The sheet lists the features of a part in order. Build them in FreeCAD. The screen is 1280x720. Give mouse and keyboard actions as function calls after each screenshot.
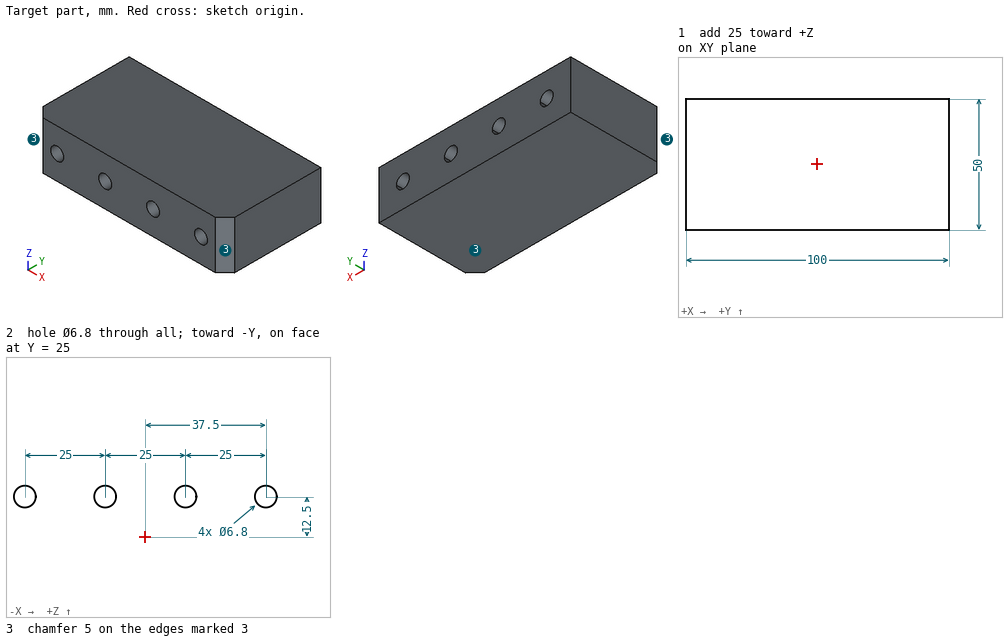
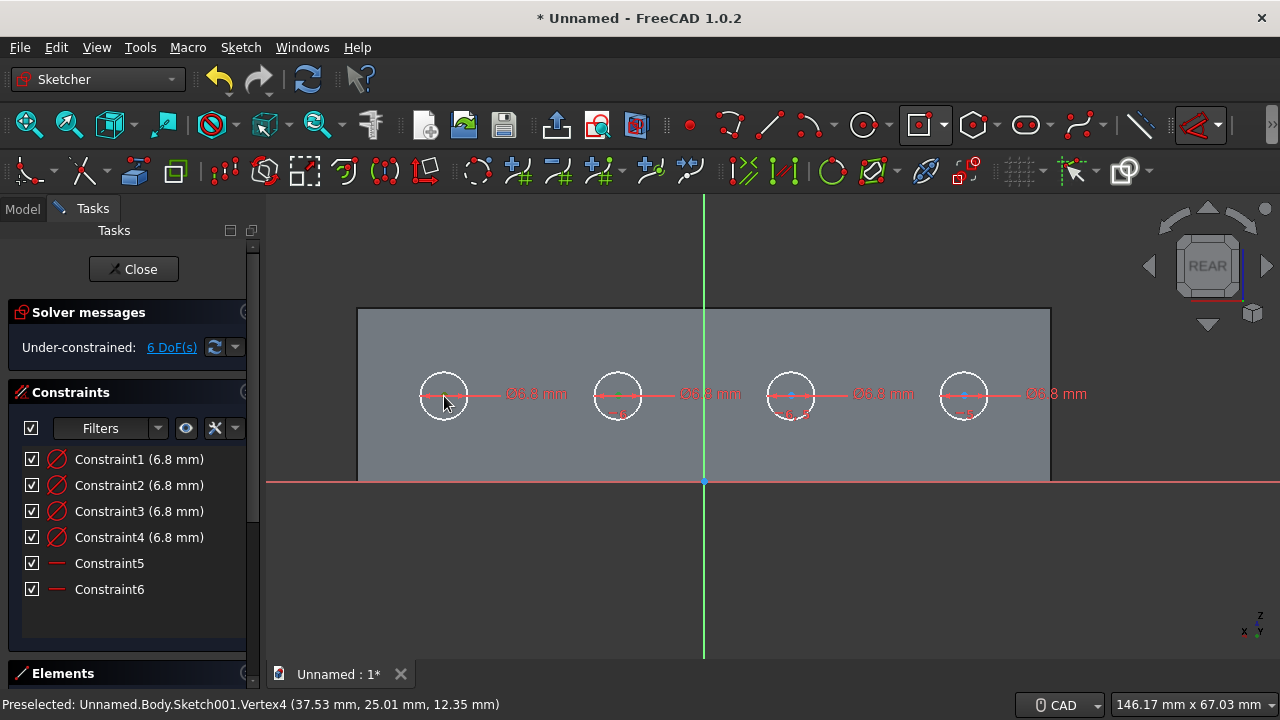
key(h)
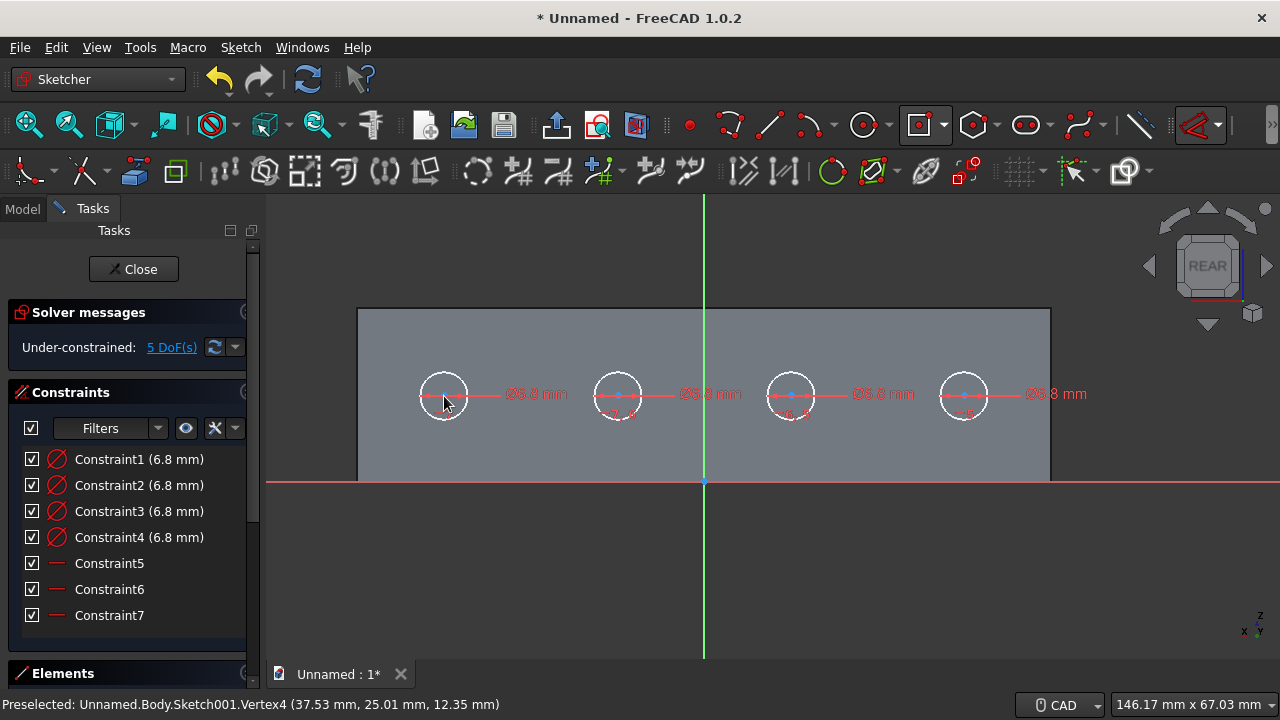
click(1194, 126)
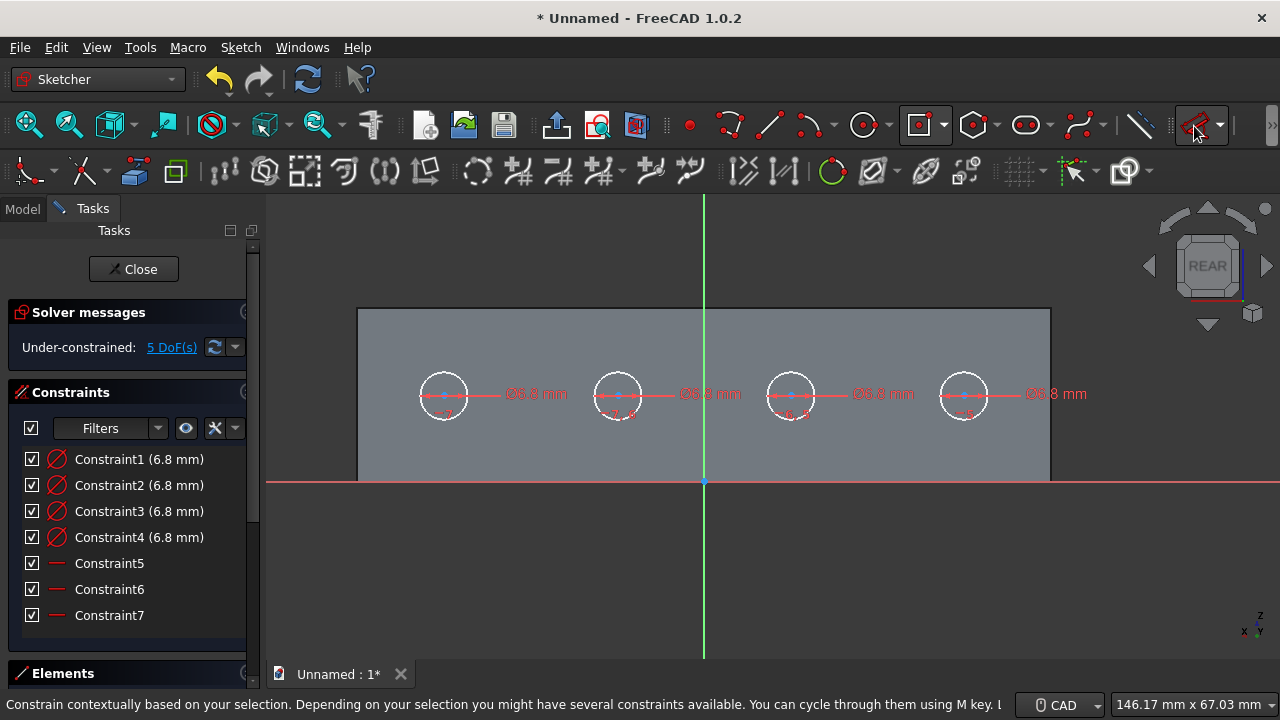
click(964, 396)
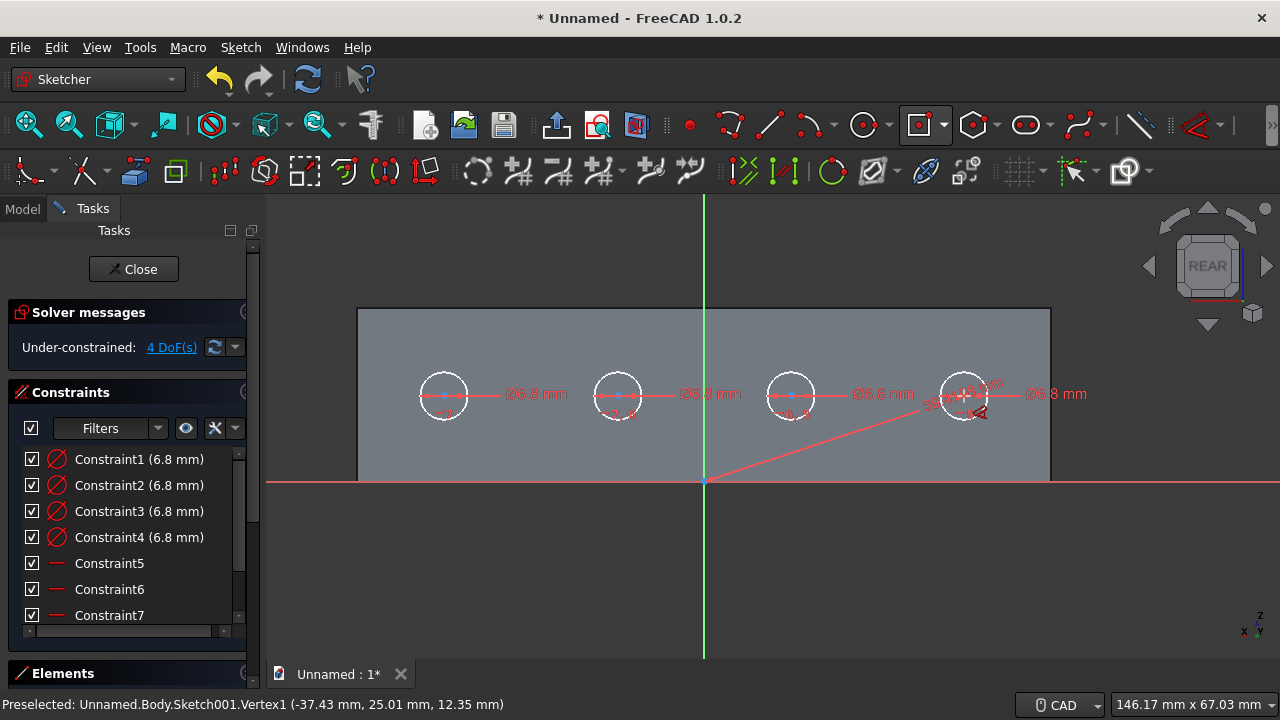
click(791, 396)
click(877, 362)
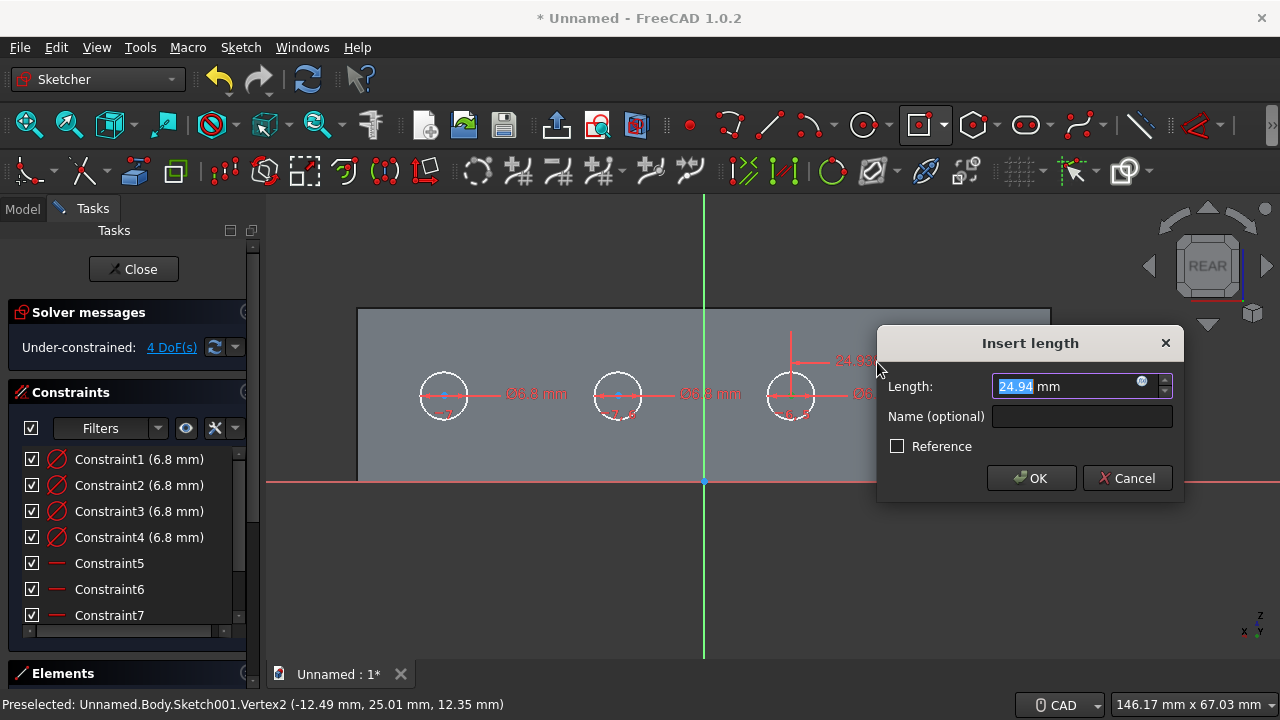
text(25)
key(Return)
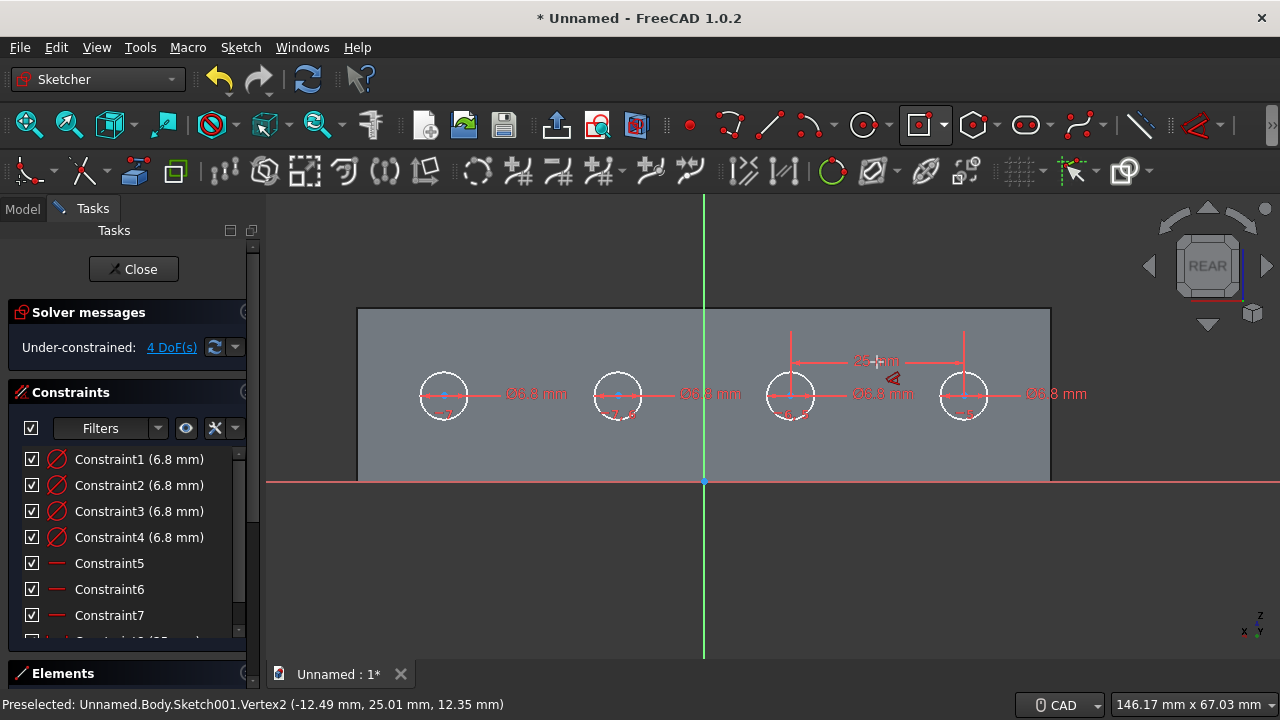
click(791, 396)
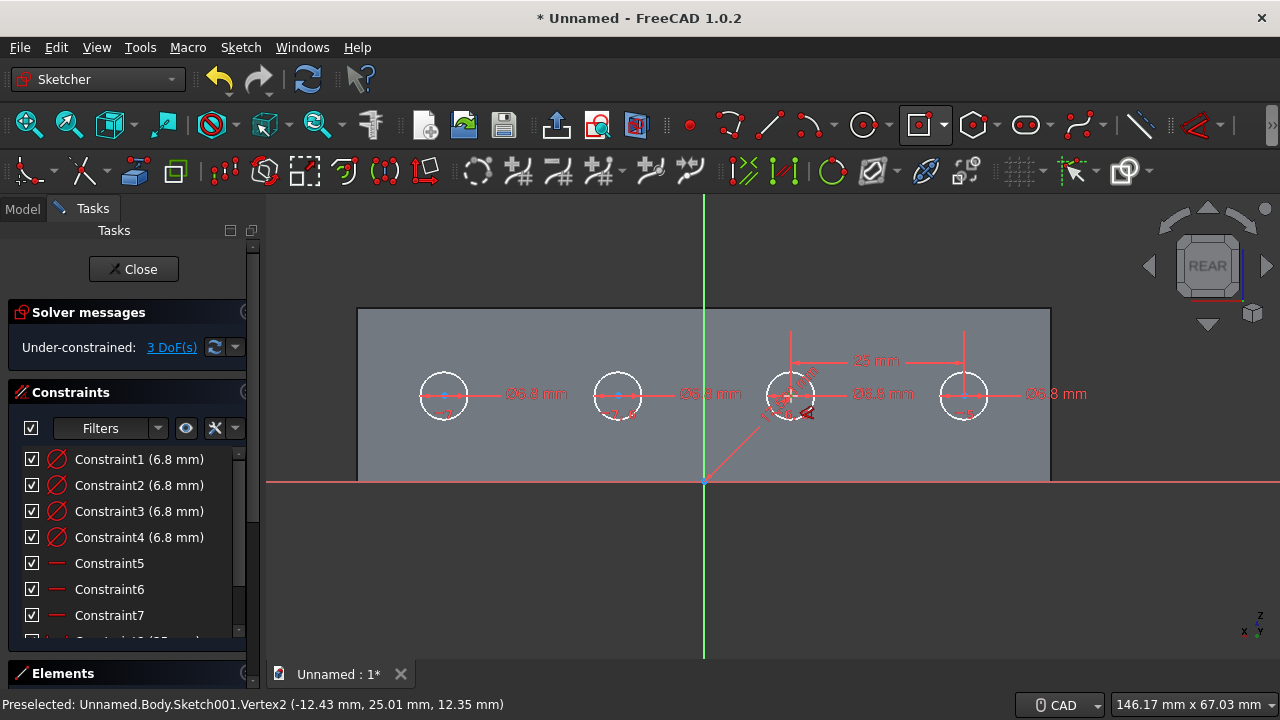
click(618, 396)
click(665, 362)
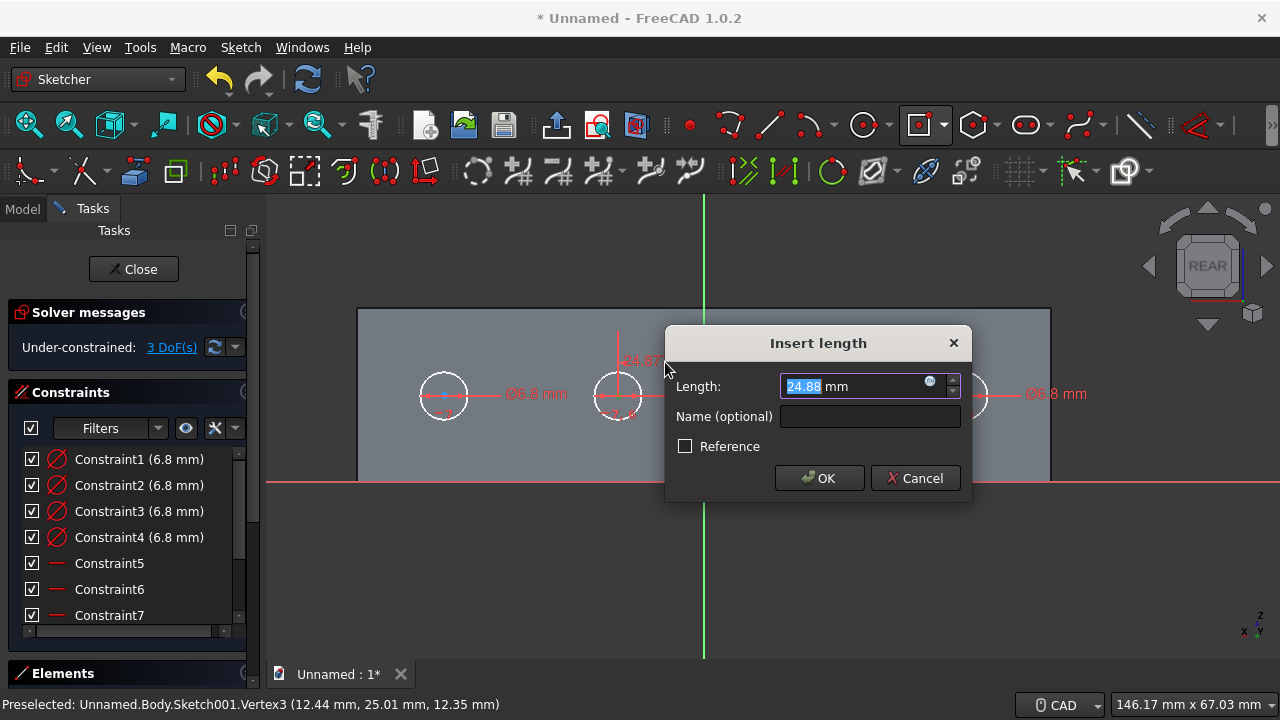
text(25)
key(Return)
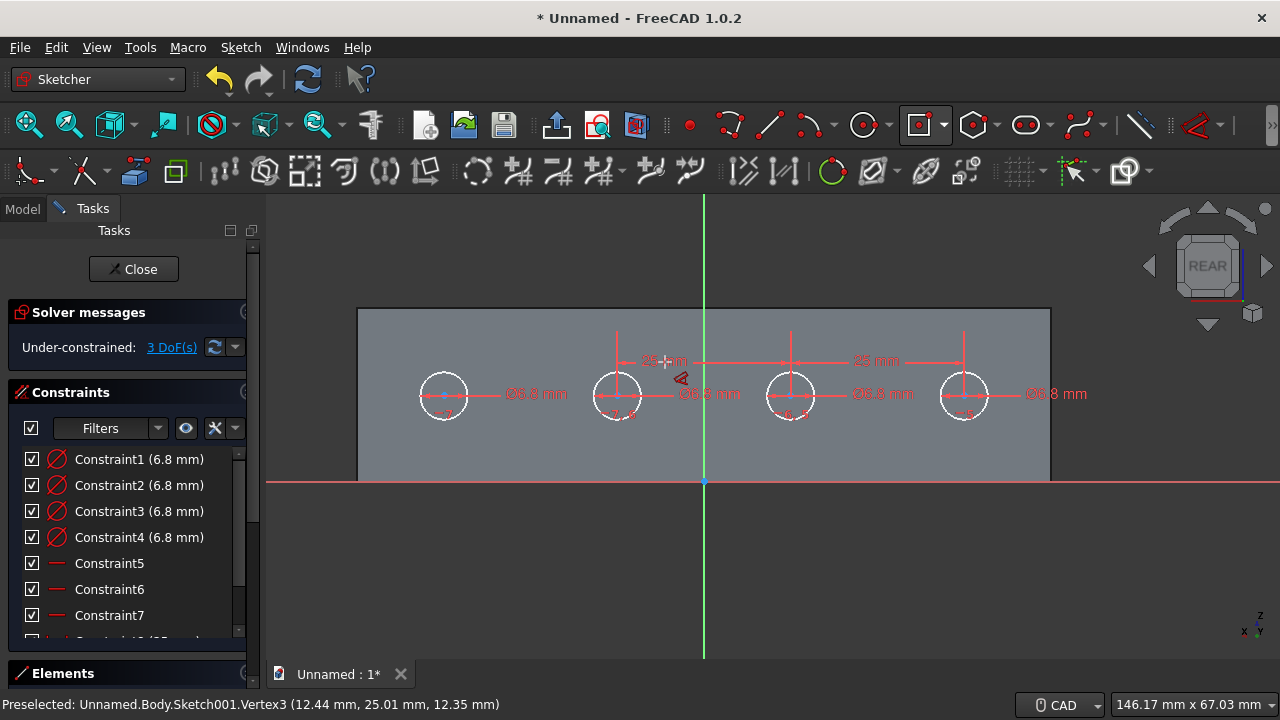
click(617, 396)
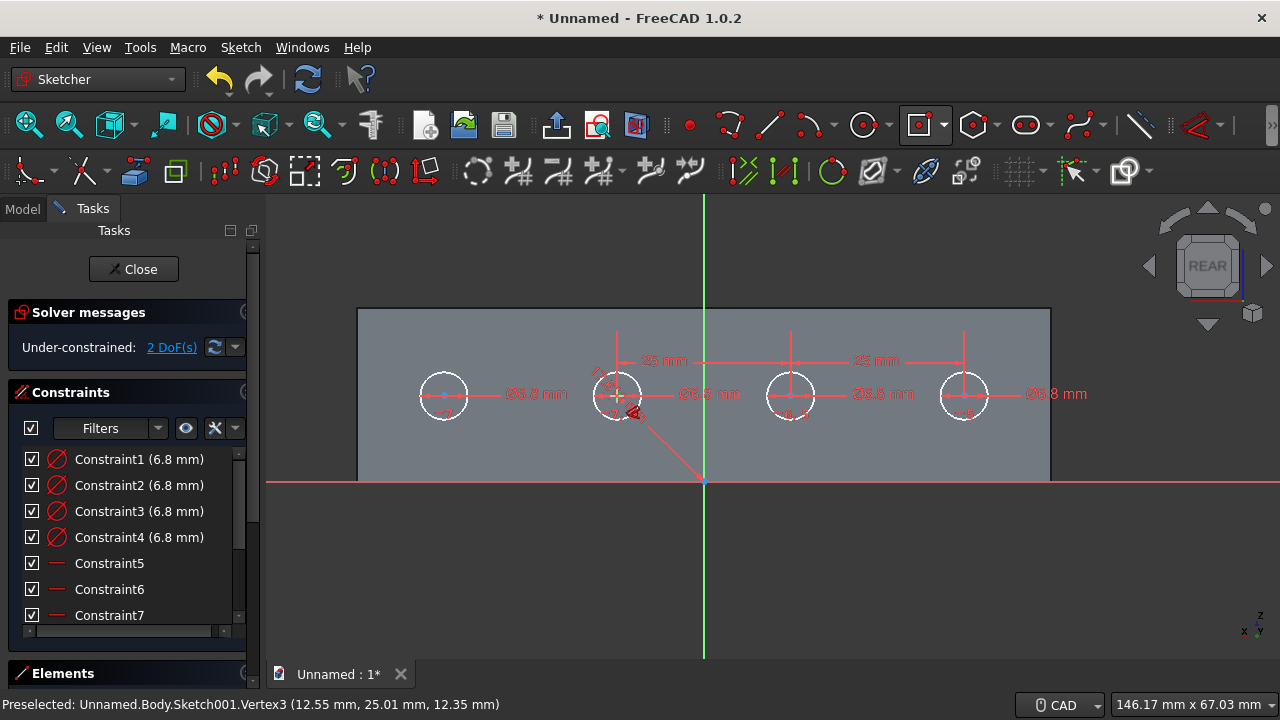
click(444, 396)
click(531, 362)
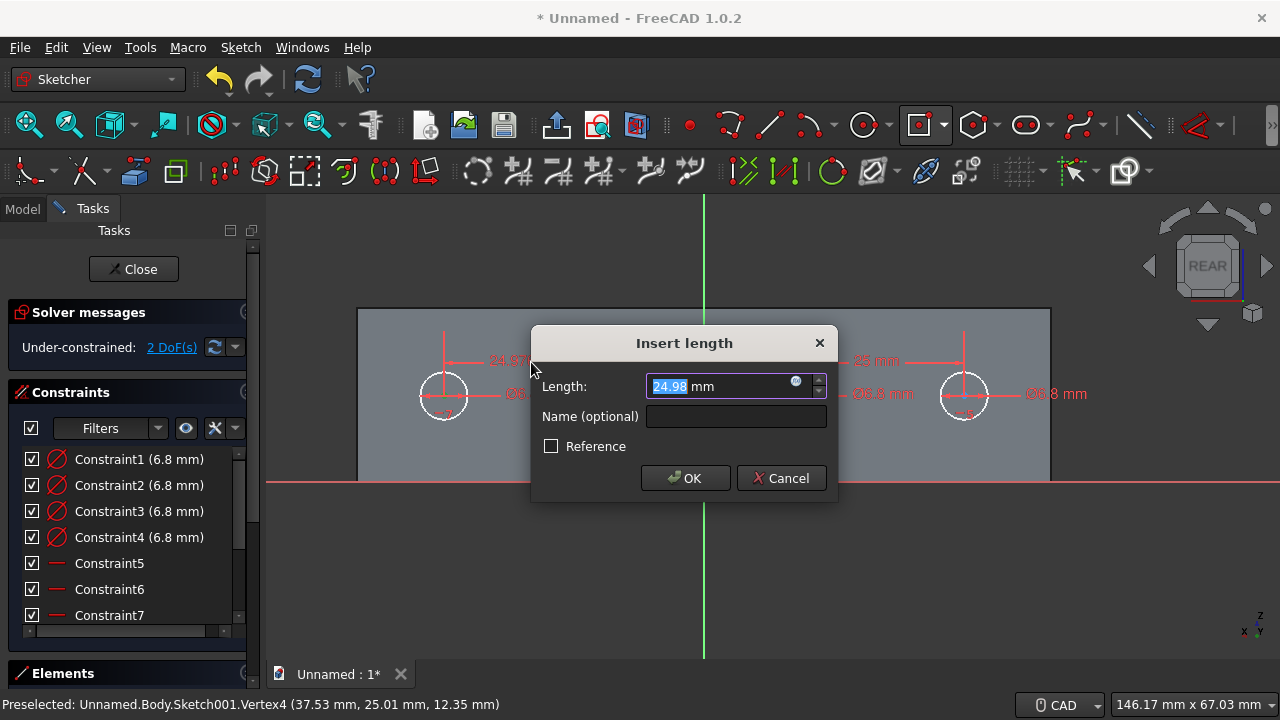
text(25)
key(Return)